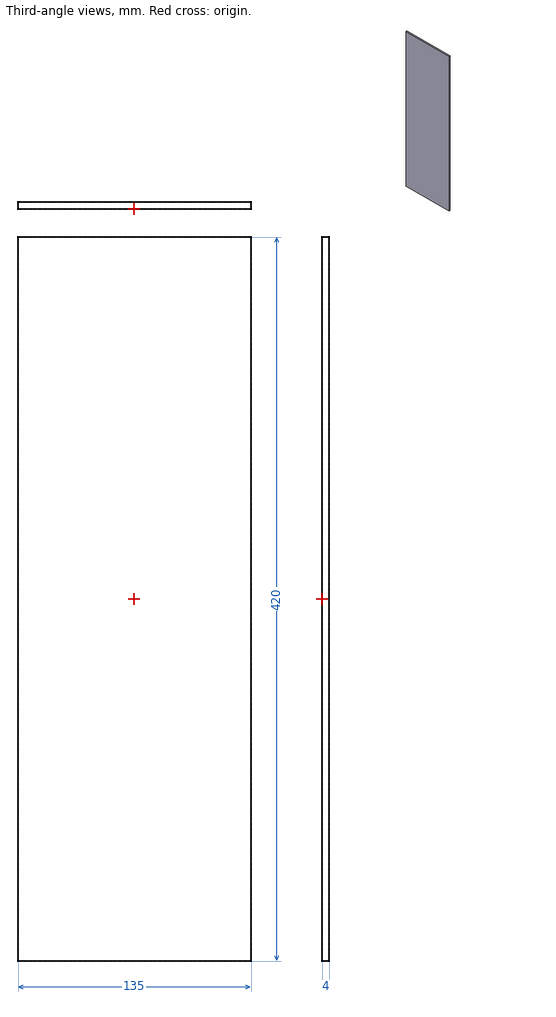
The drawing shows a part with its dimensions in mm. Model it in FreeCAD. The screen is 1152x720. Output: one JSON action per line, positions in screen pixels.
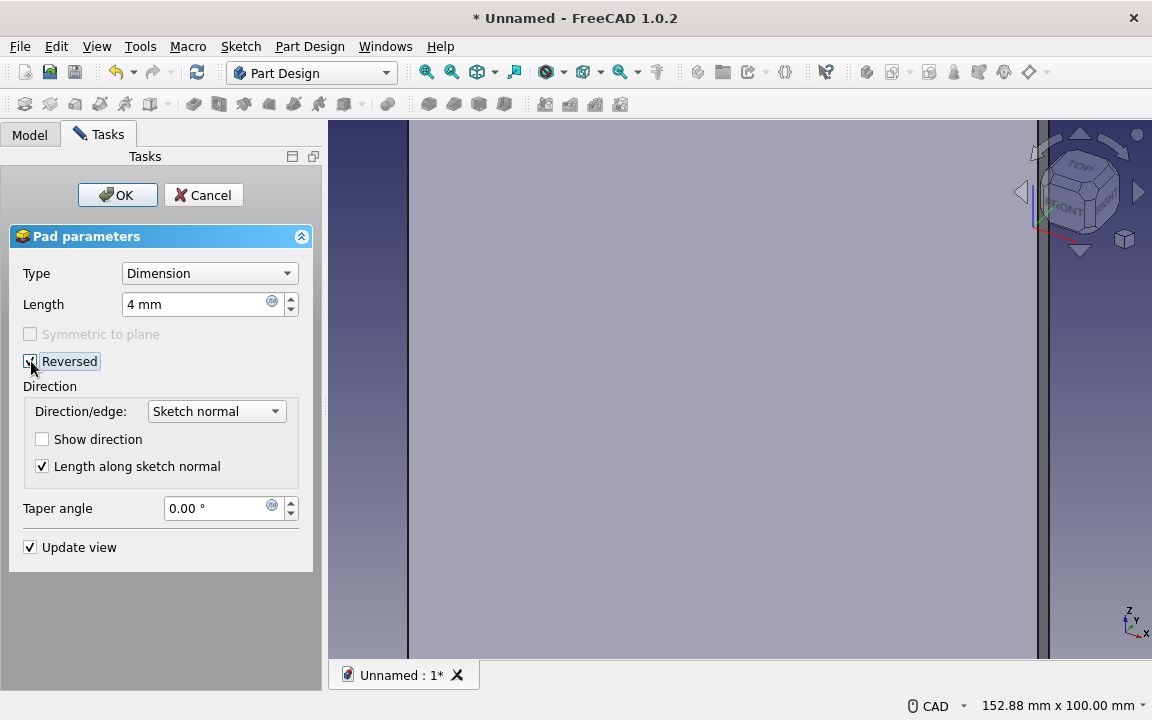
{"action": "left_click", "coordinate": [118, 195]}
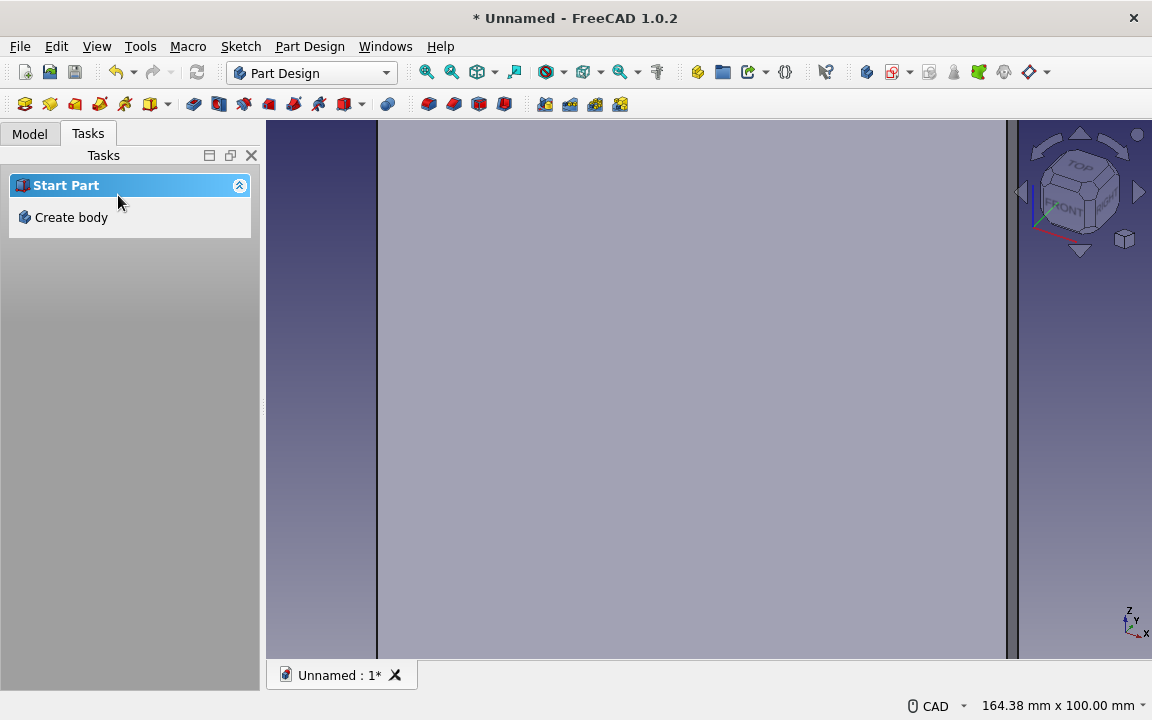
{"action": "key", "text": "0"}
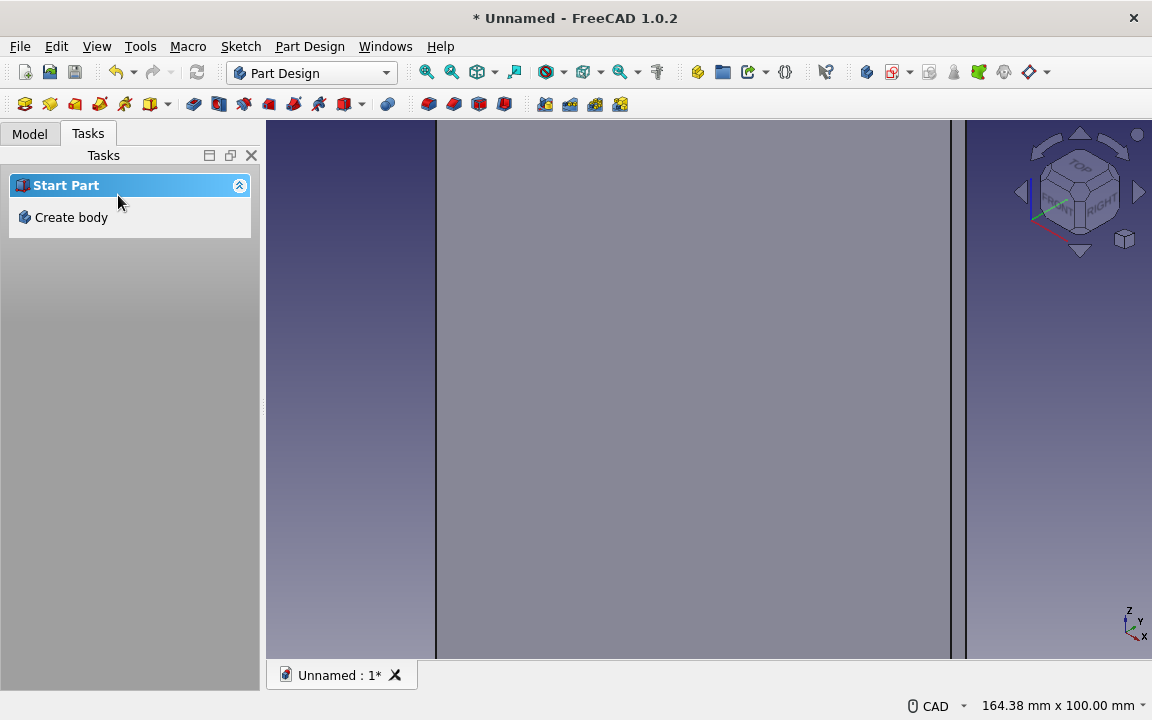
{"action": "left_click", "coordinate": [427, 72]}